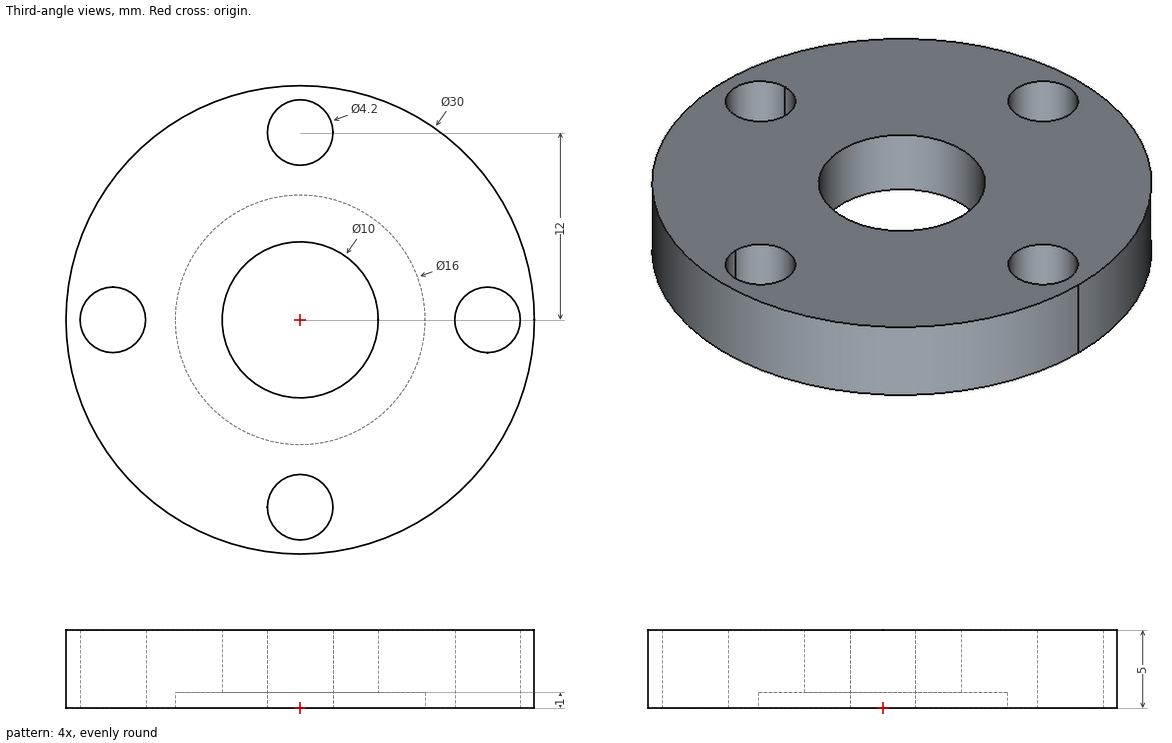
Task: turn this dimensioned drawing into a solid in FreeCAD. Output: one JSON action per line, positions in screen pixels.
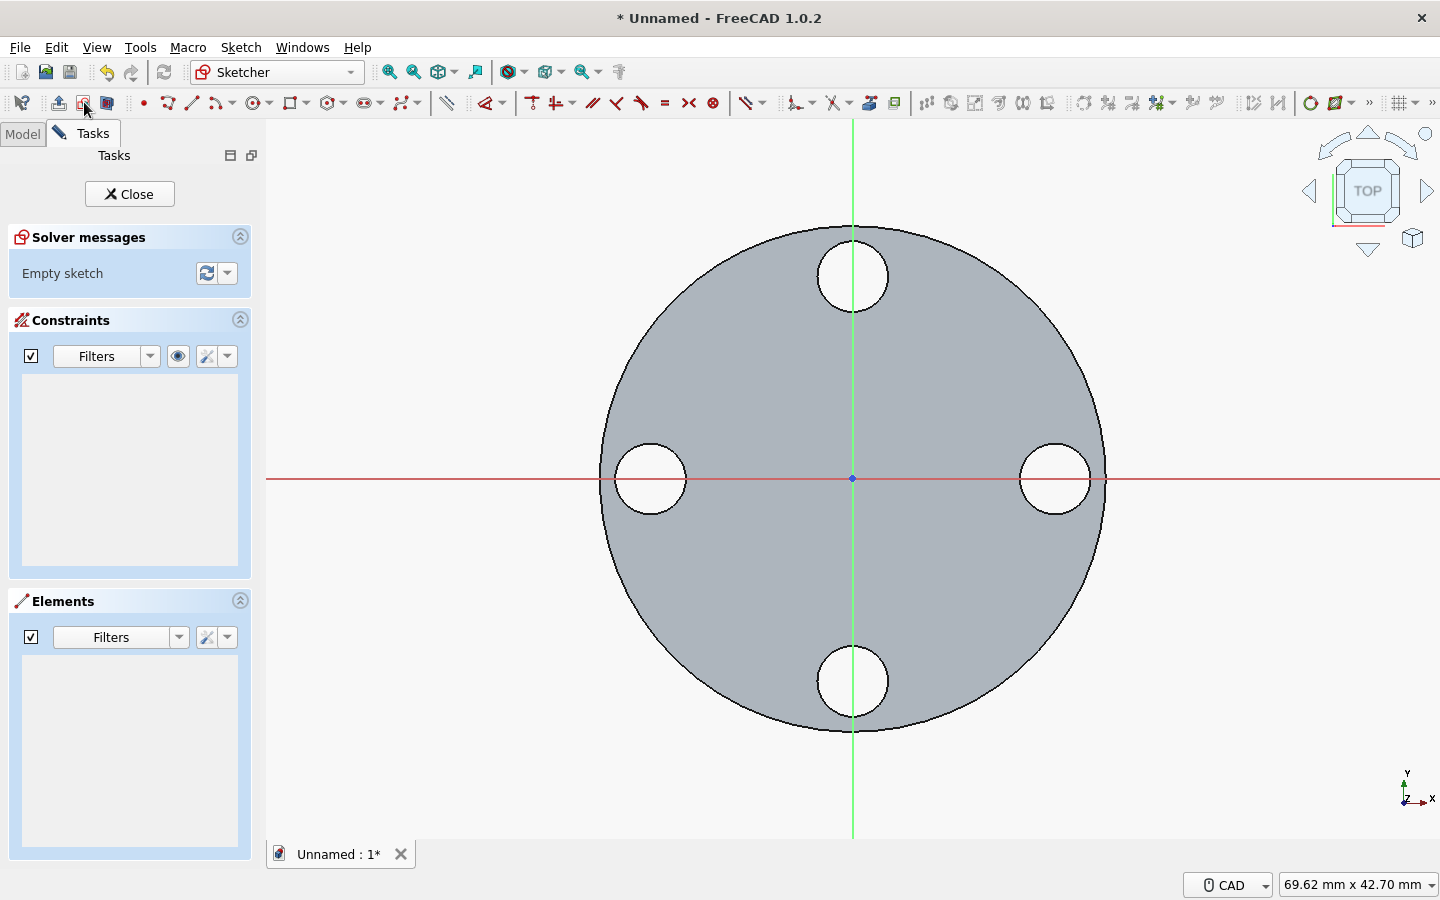
{"action": "scroll", "coordinate": [893, 479], "scroll_direction": "up", "scroll_amount": 5}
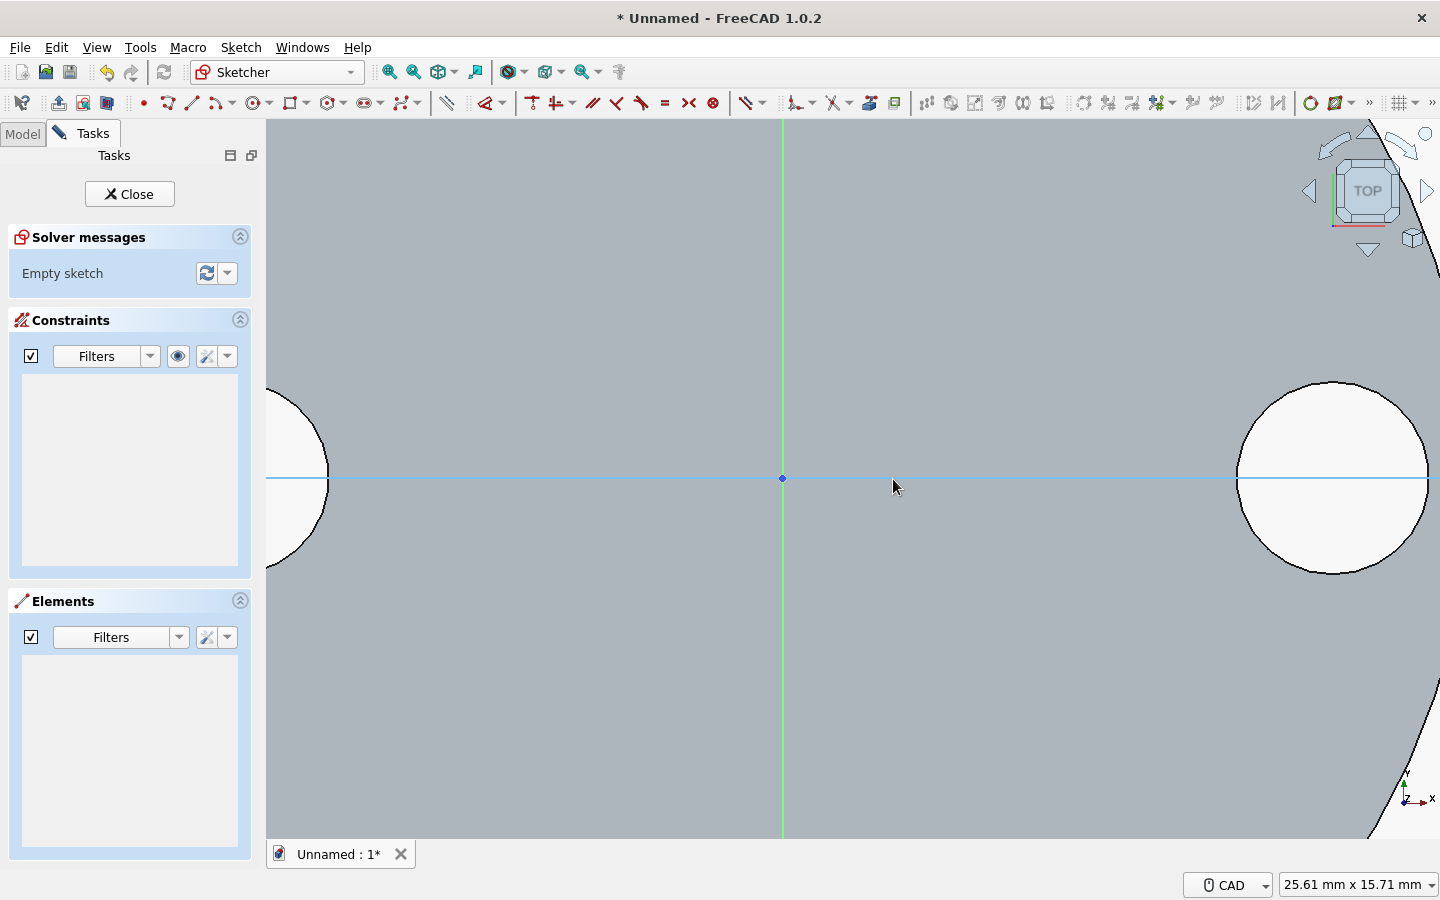
{"action": "left_click", "coordinate": [254, 104]}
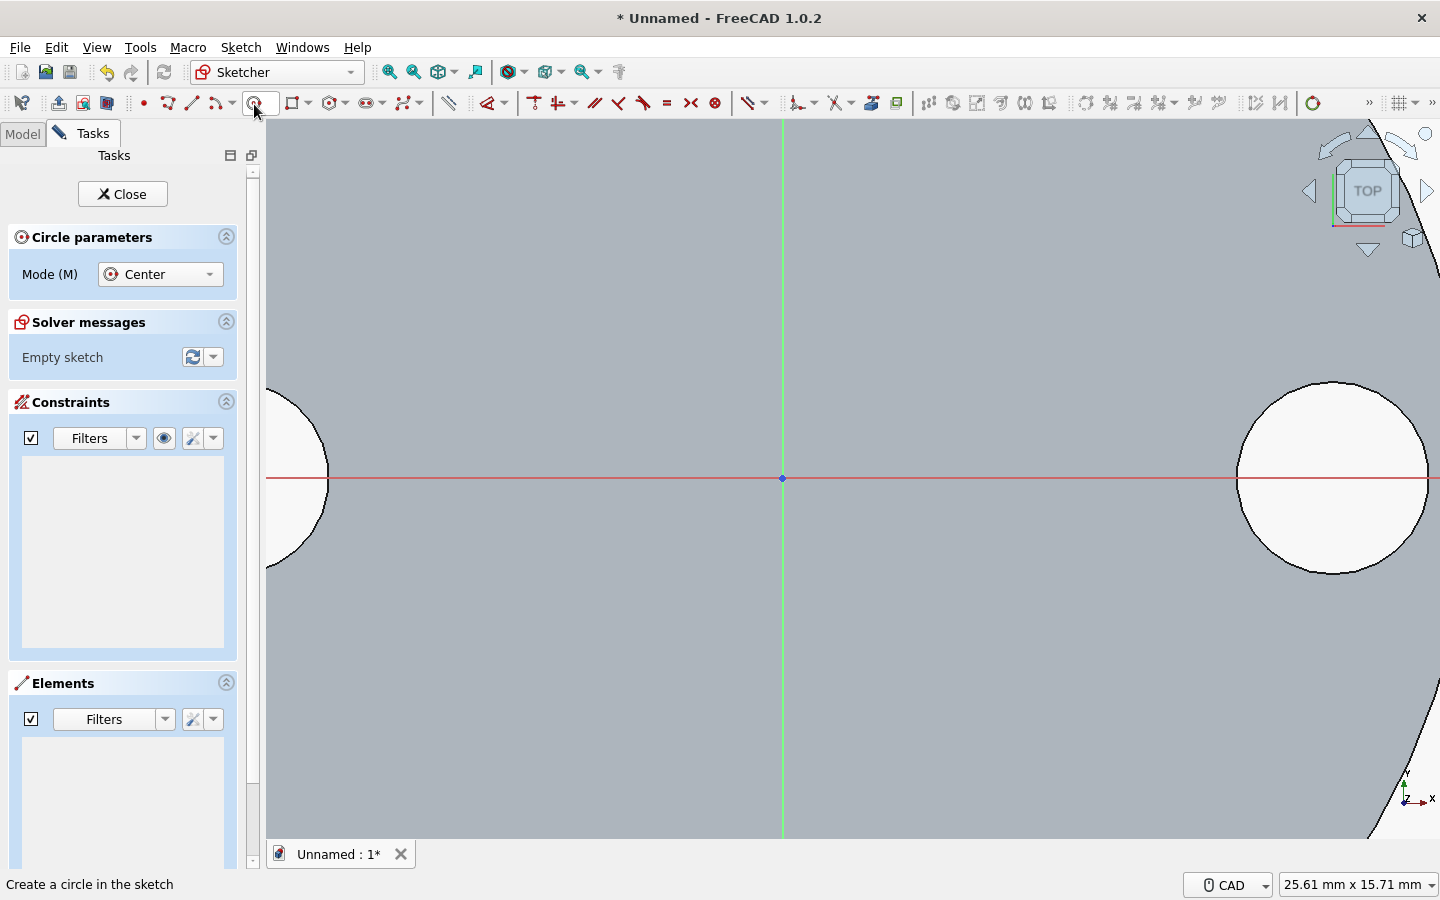
{"action": "left_click", "coordinate": [783, 478]}
{"action": "mouse_move", "coordinate": [945, 316]}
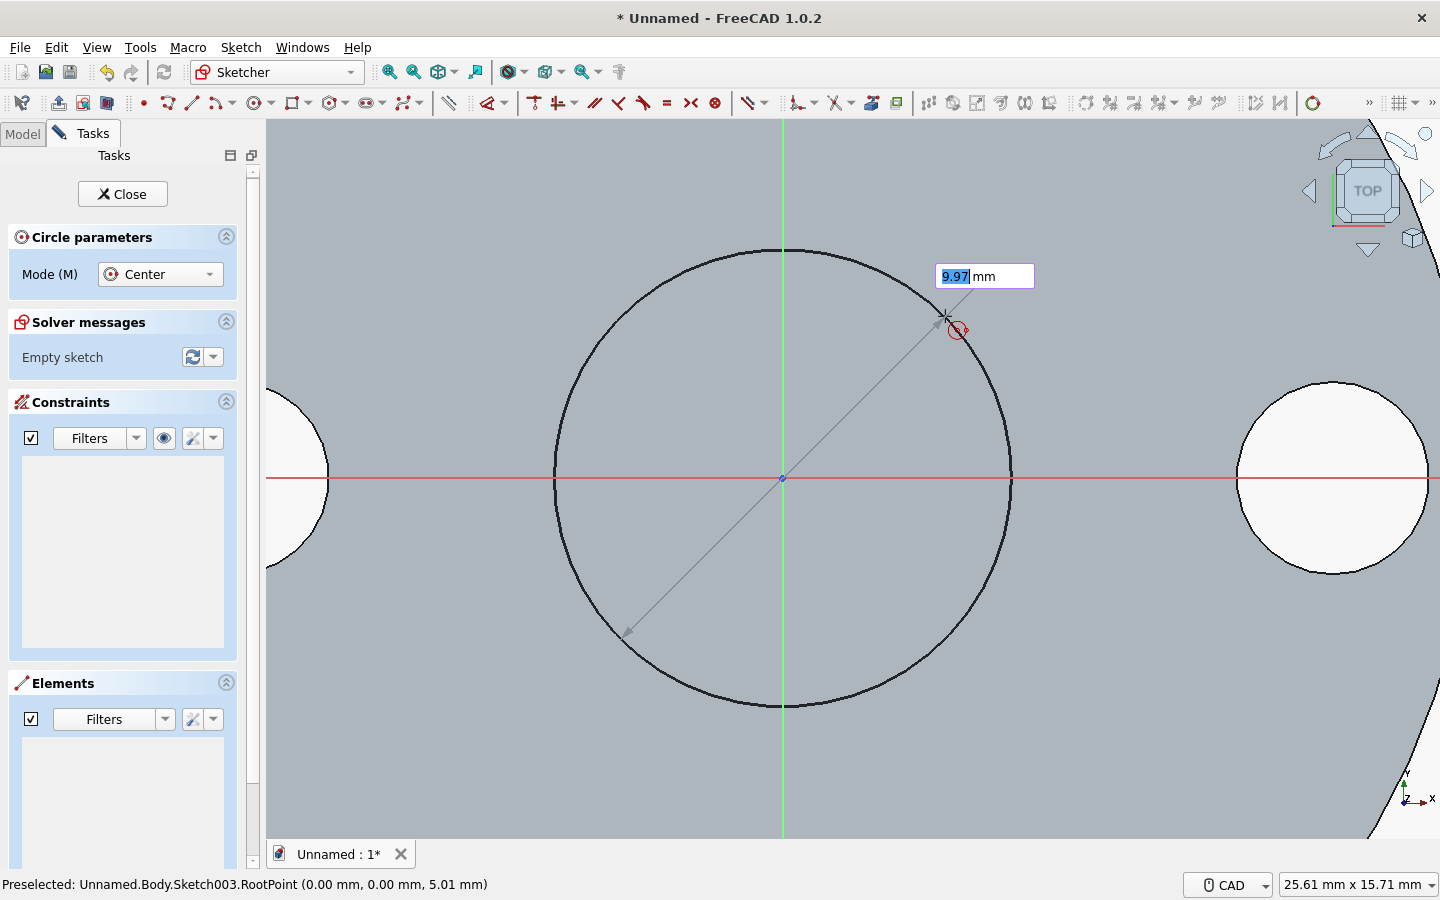
{"action": "type", "text": "10"}
{"action": "key", "text": "Return"}
{"action": "key", "text": "Escape"}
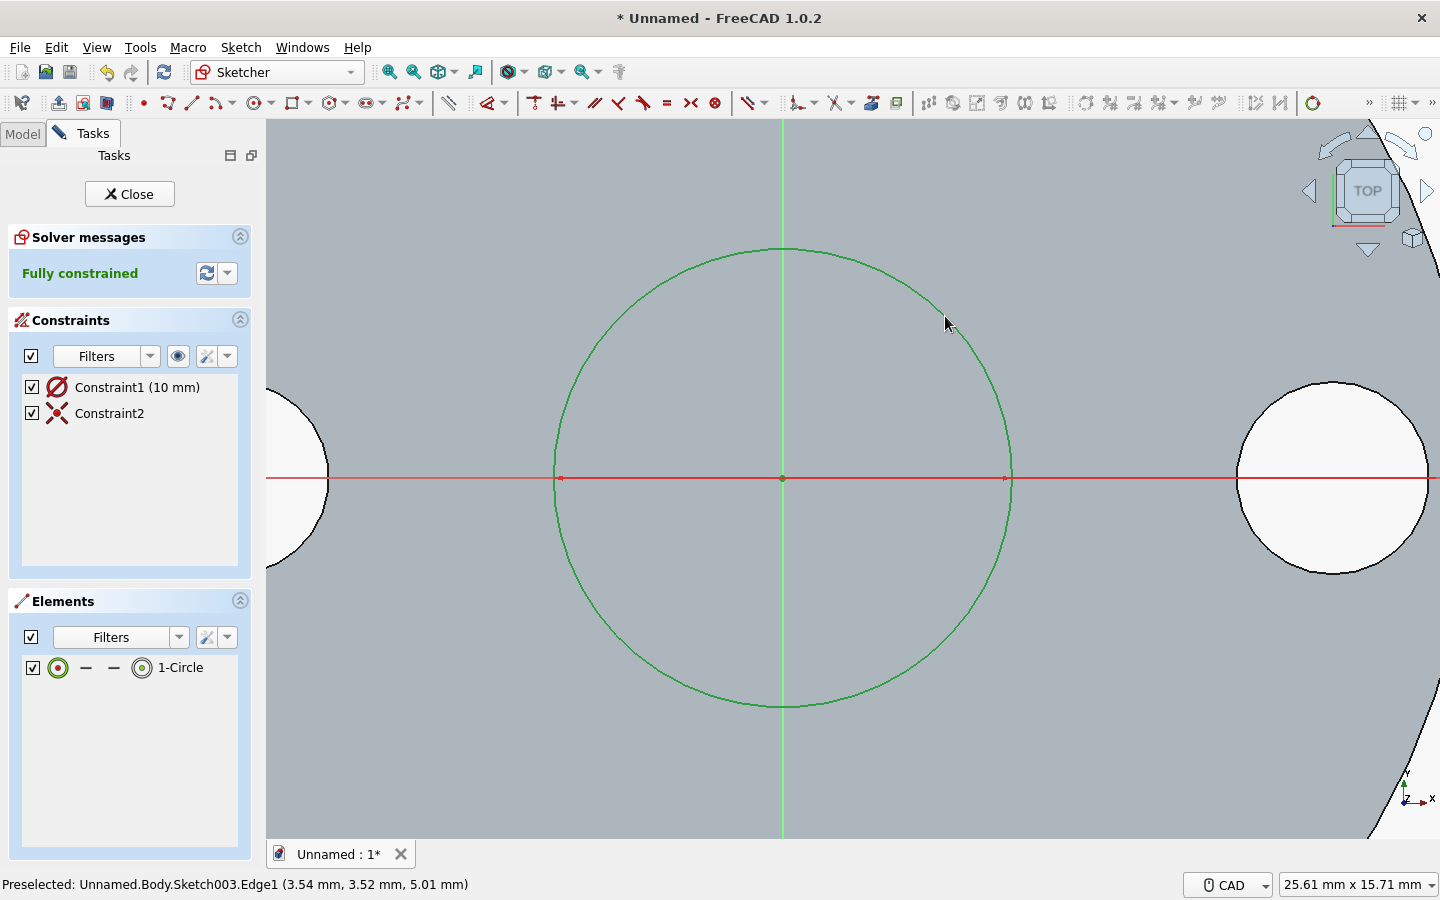
{"action": "left_click", "coordinate": [130, 194]}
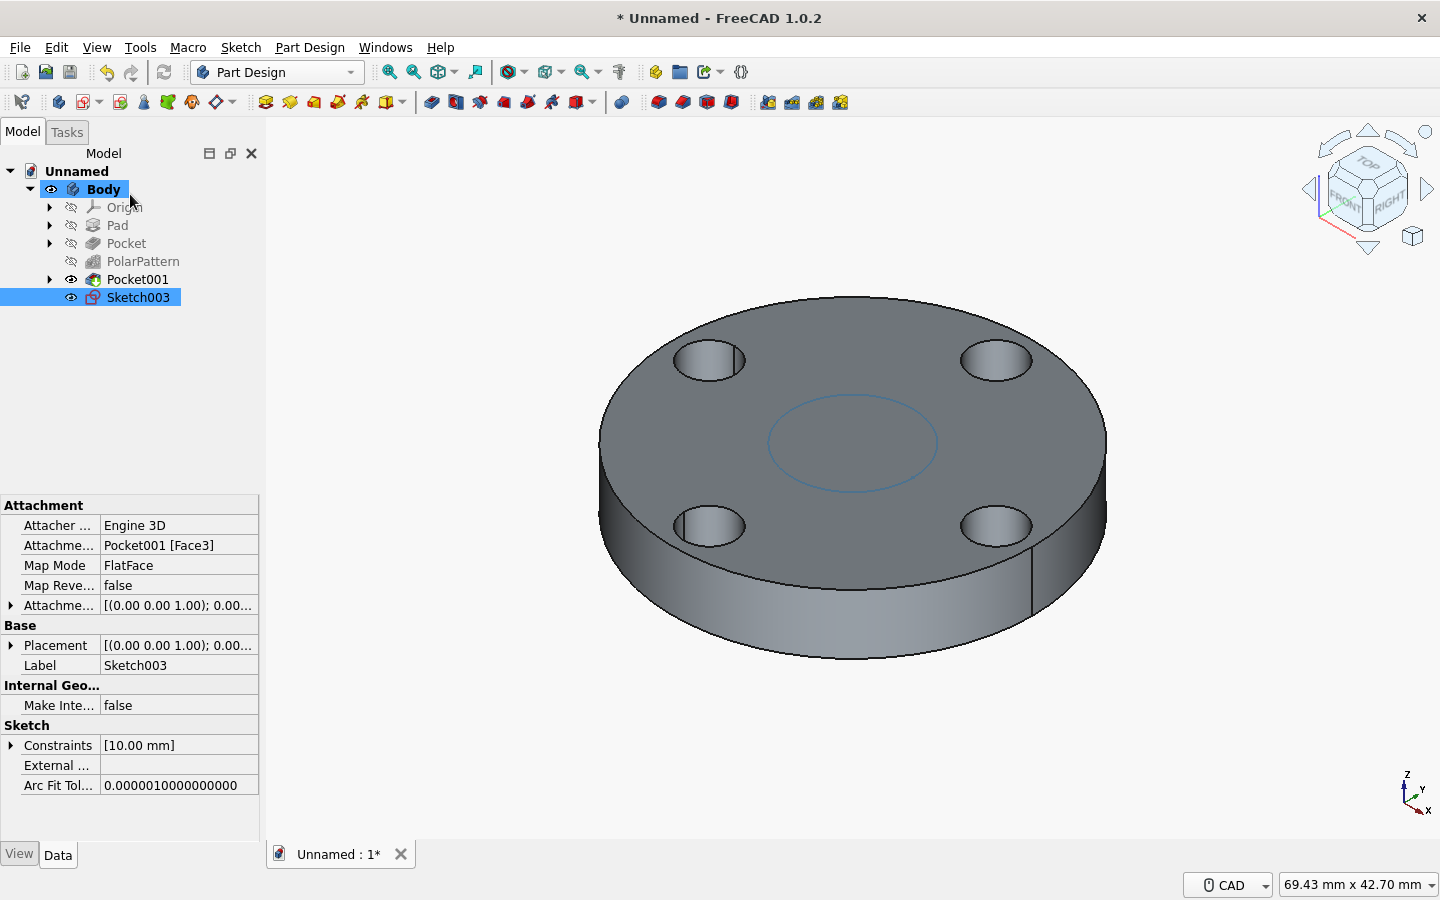
{"action": "left_click", "coordinate": [432, 102]}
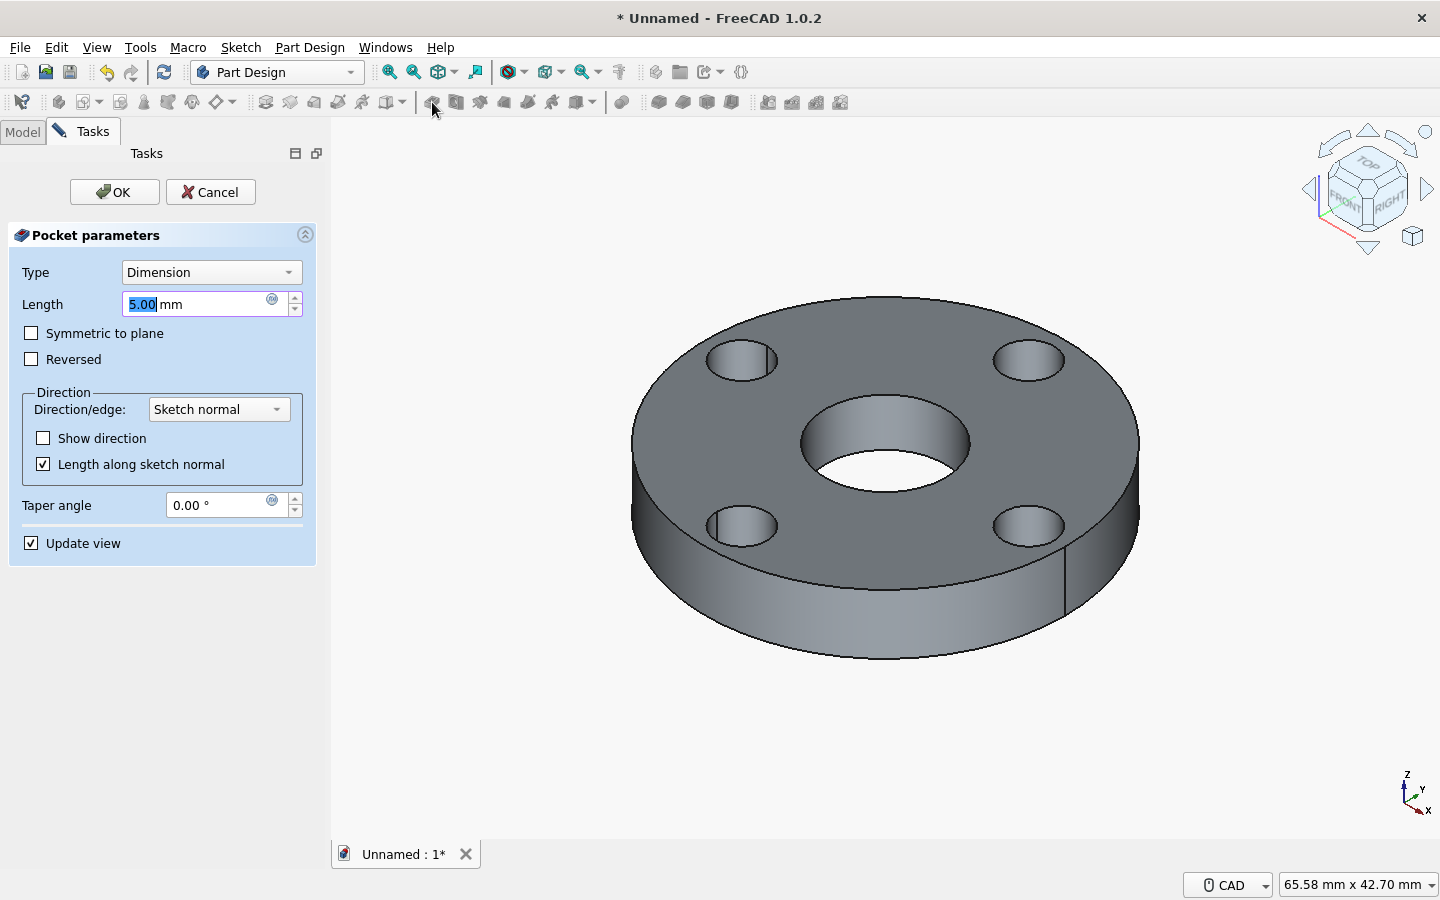
{"action": "left_click", "coordinate": [212, 272]}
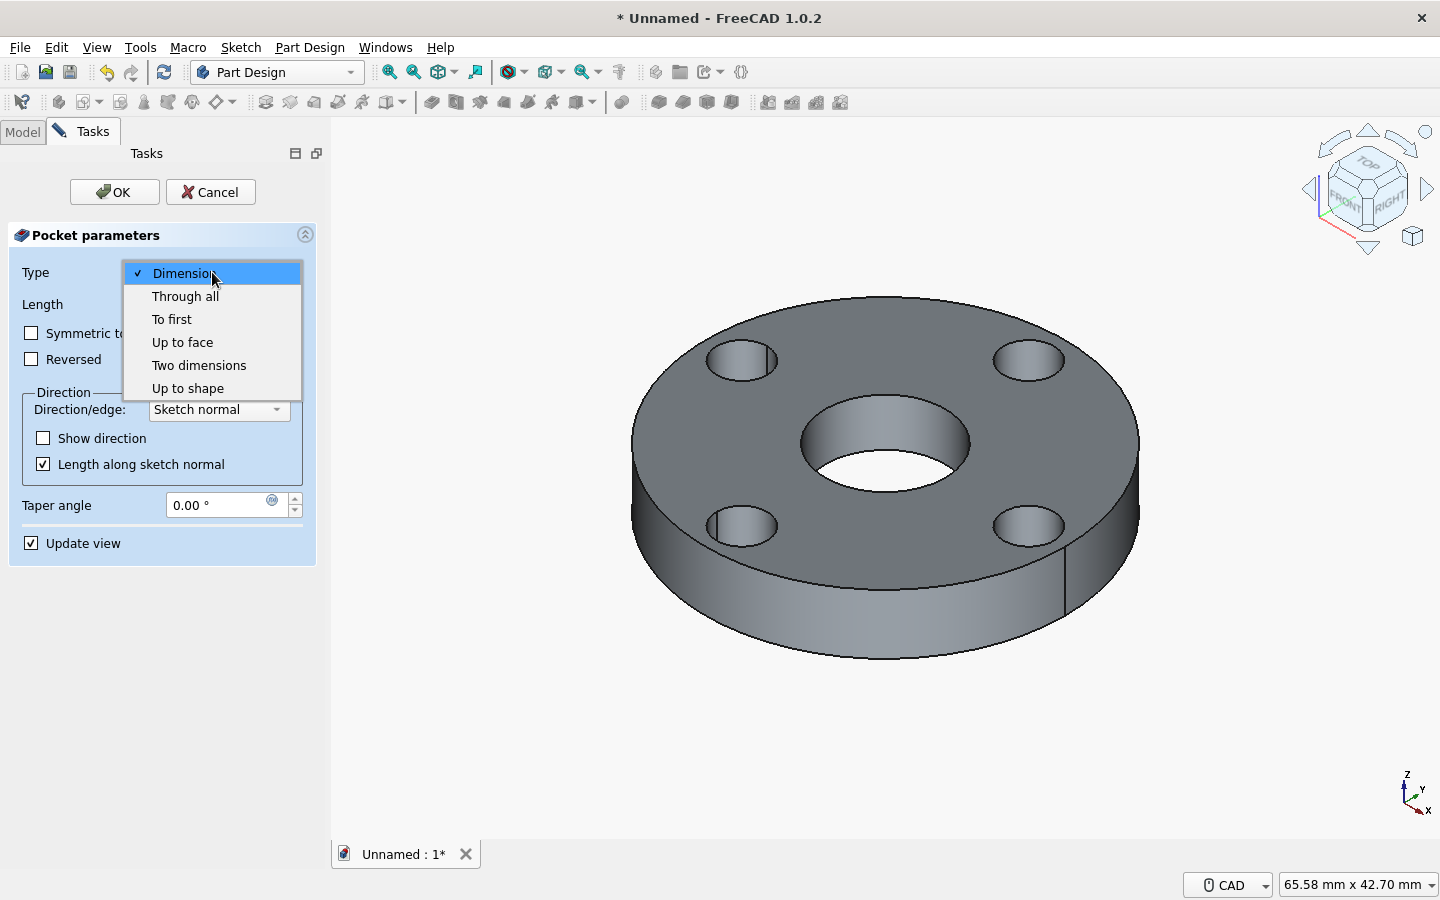
{"action": "left_click", "coordinate": [212, 296]}